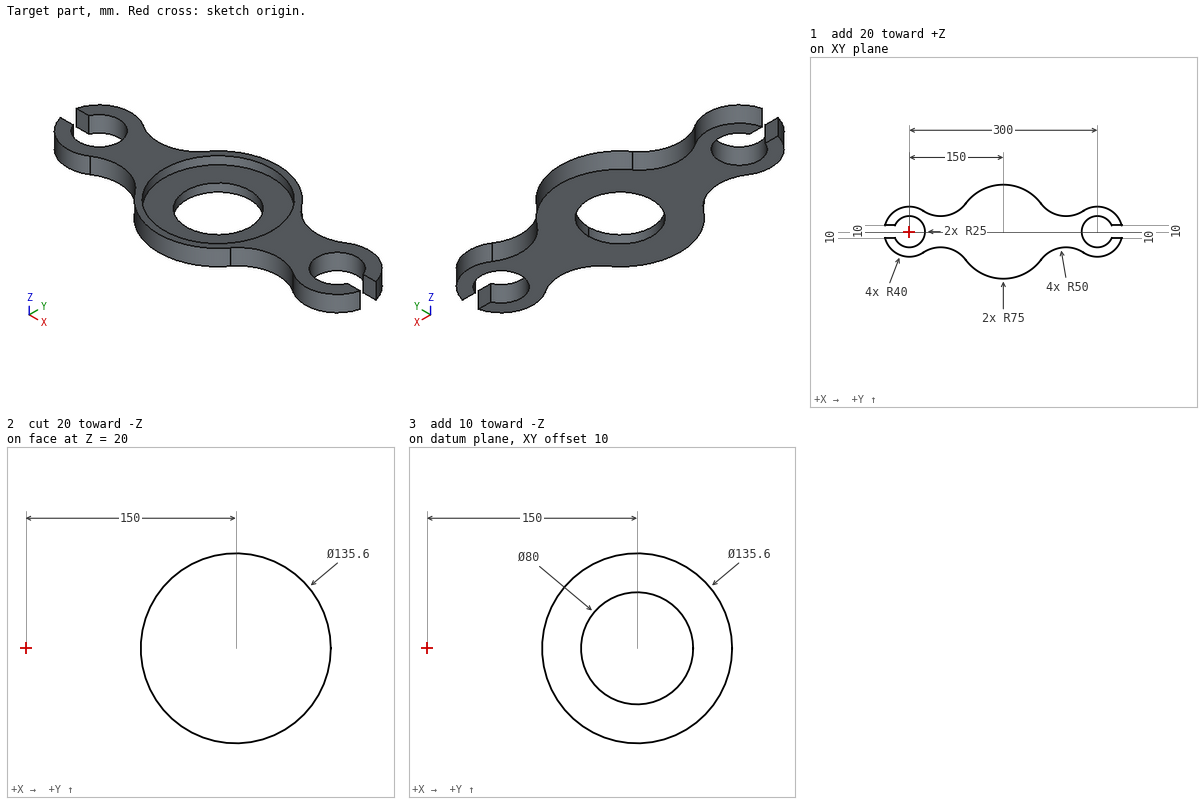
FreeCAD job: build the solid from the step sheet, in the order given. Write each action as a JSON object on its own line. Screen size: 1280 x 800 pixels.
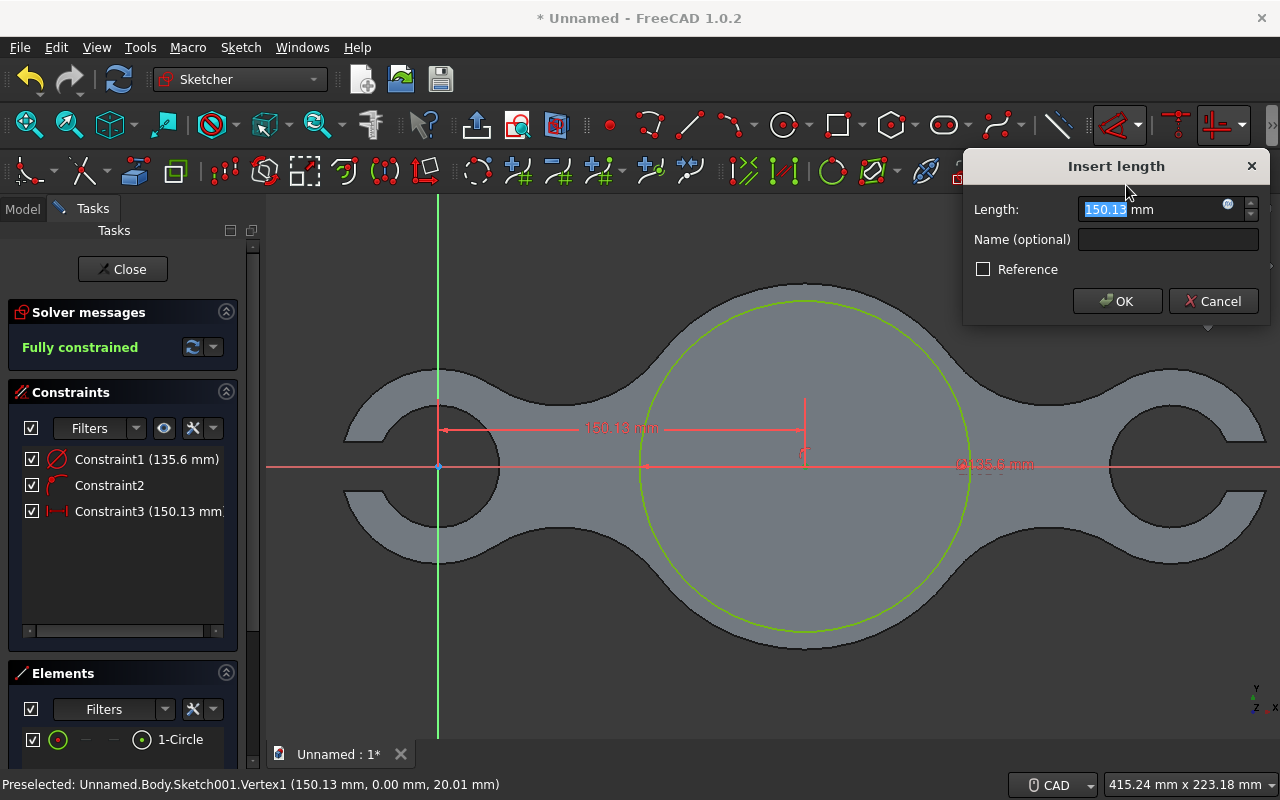
{"action": "type", "text": "150"}
{"action": "key", "text": "Return"}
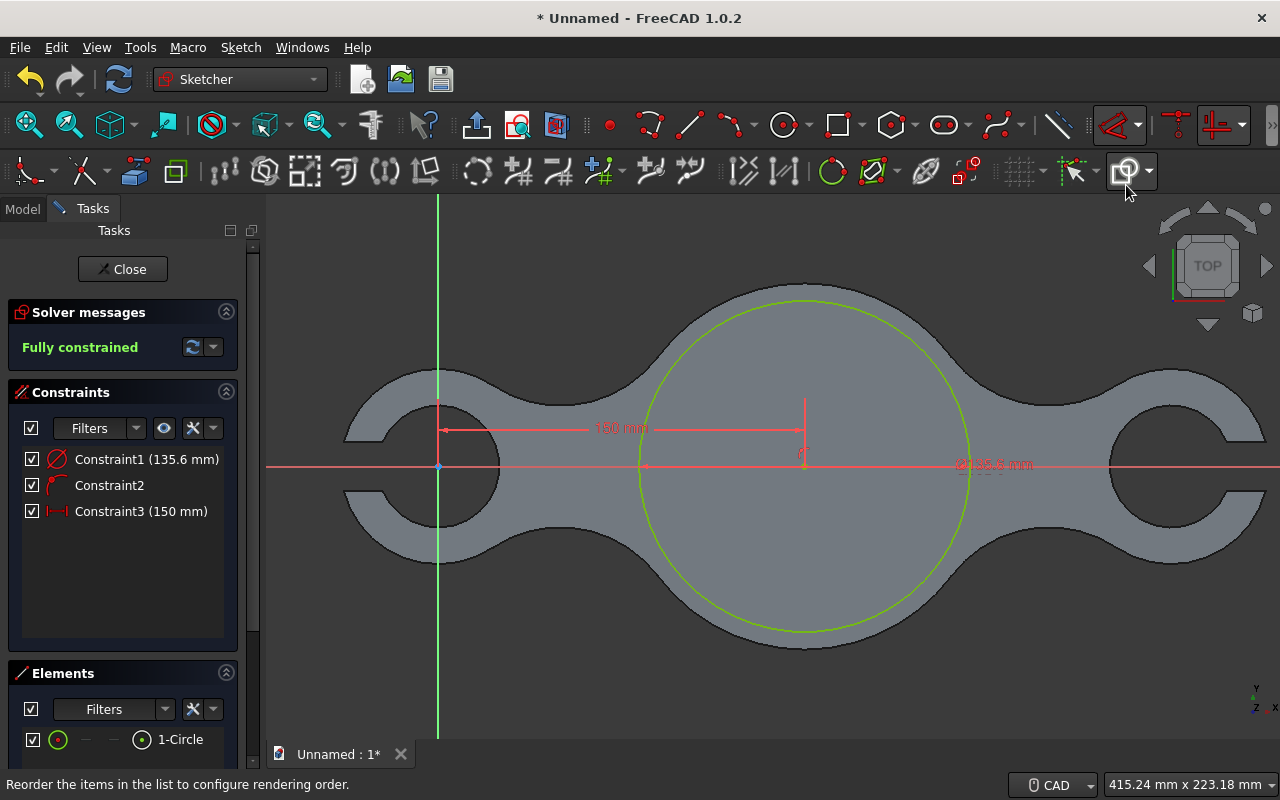
{"action": "left_click", "coordinate": [123, 269]}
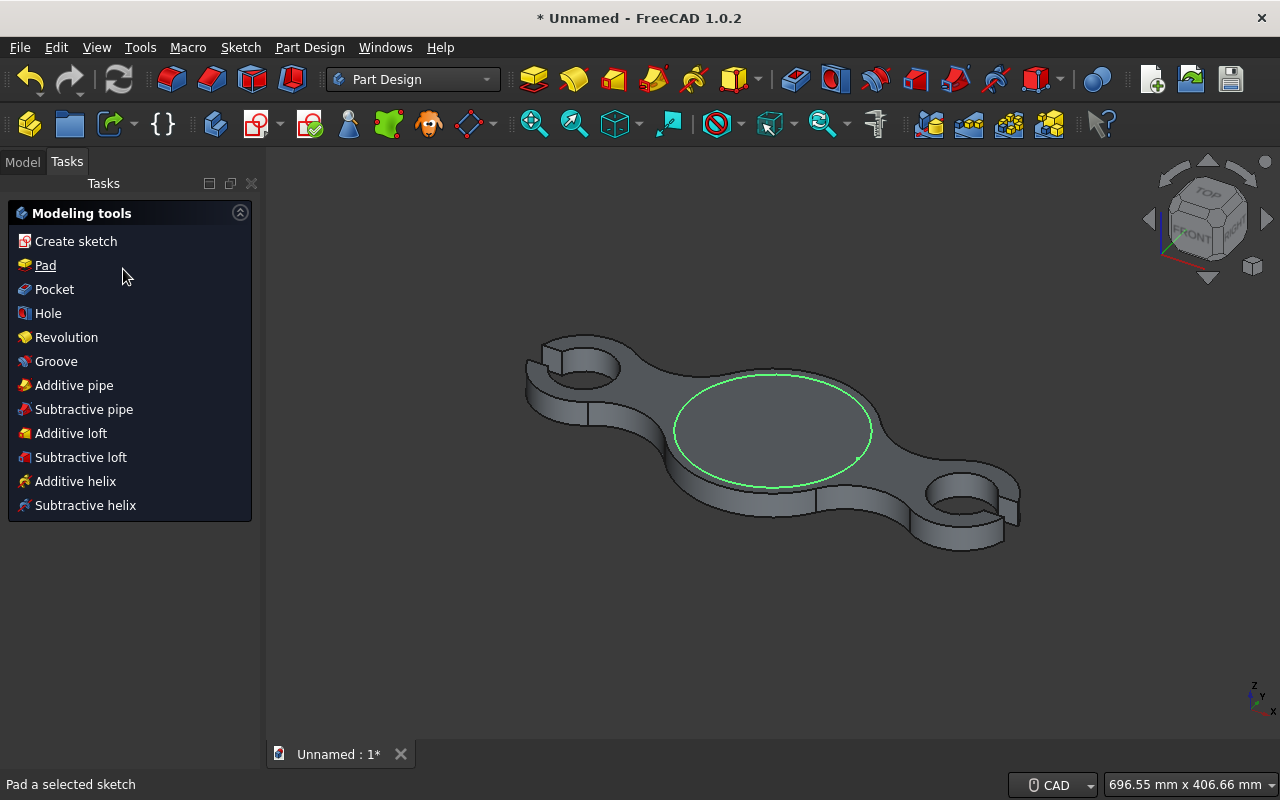
{"action": "left_click", "coordinate": [796, 80]}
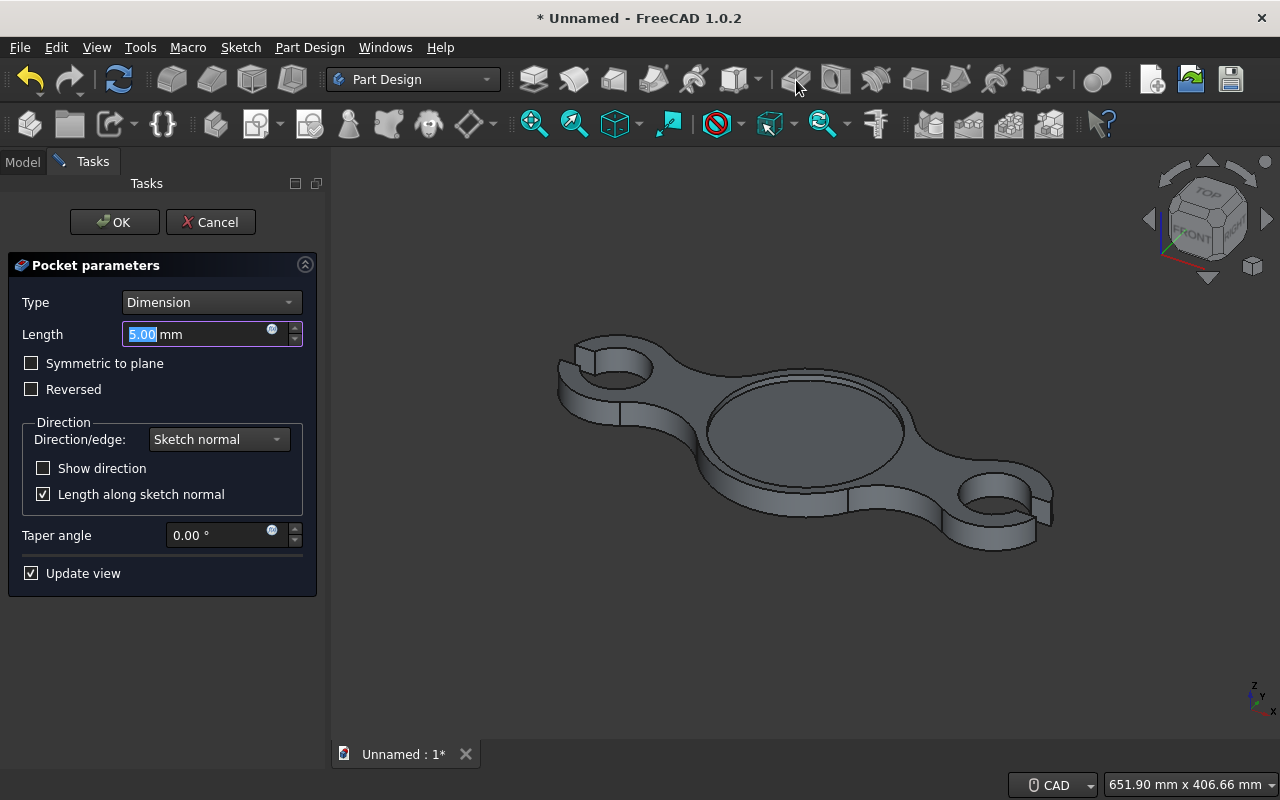
{"action": "type", "text": "20"}
{"action": "key", "text": "Tab"}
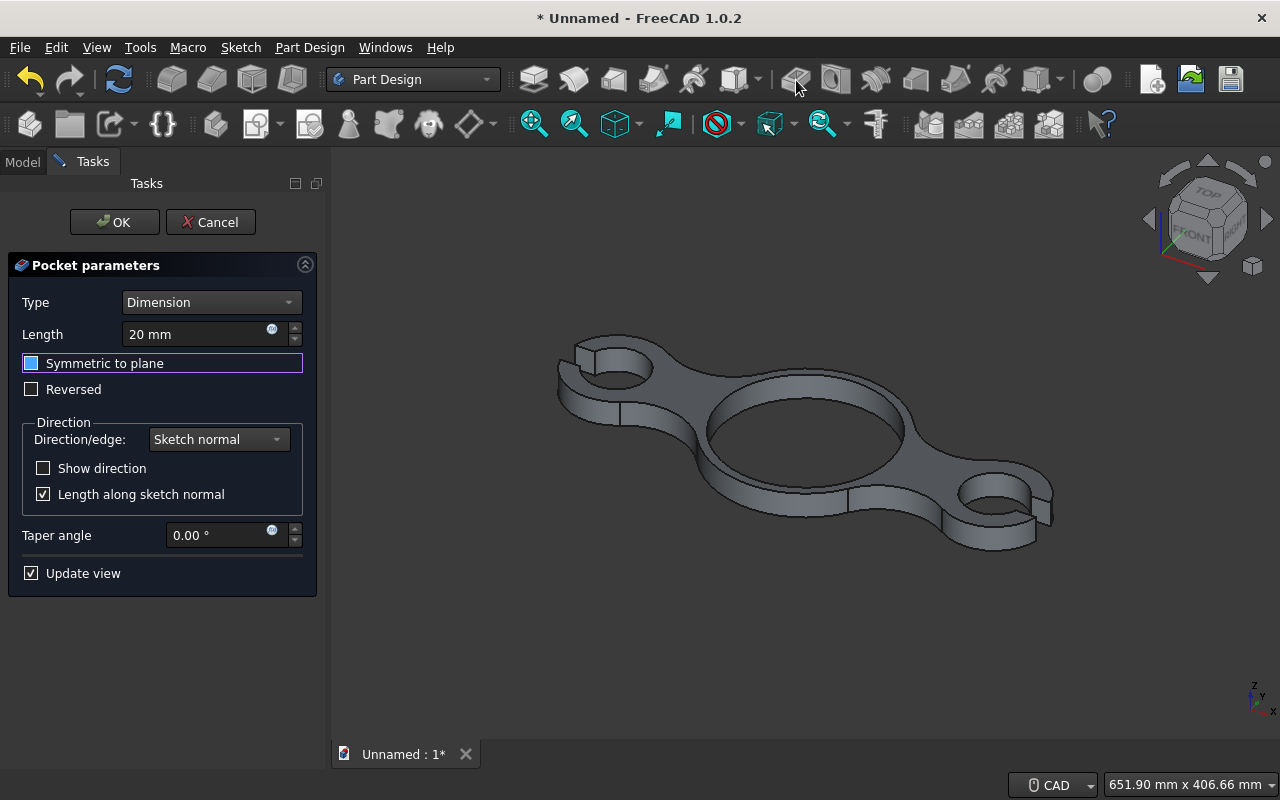
{"action": "left_click", "coordinate": [115, 222]}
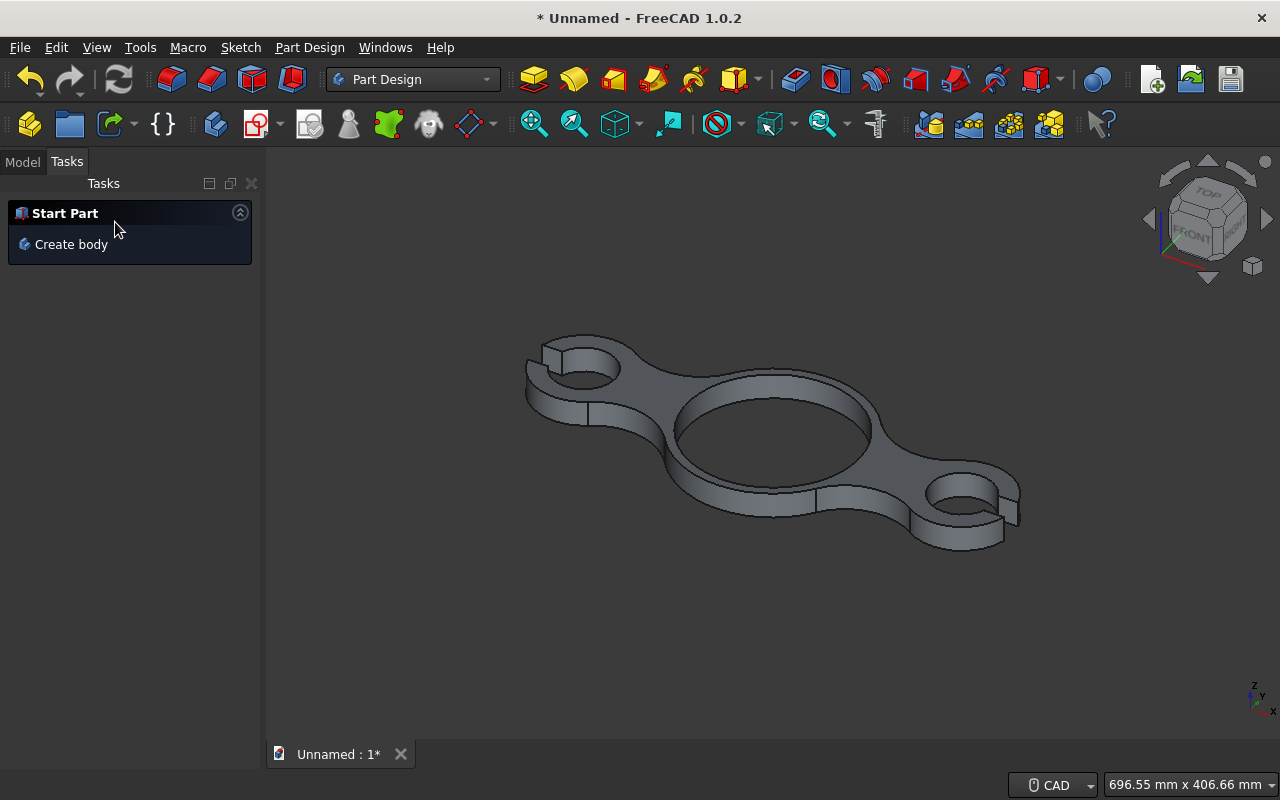
{"action": "left_click", "coordinate": [23, 161]}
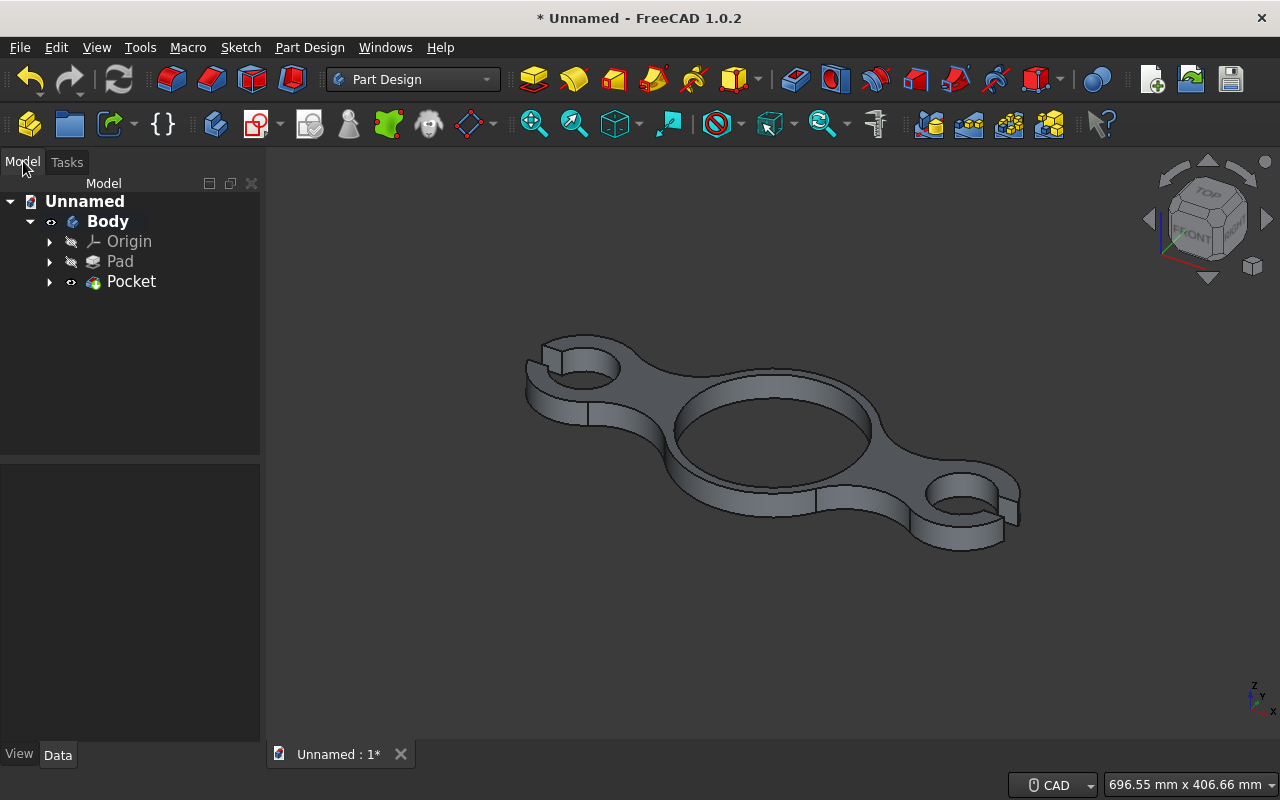
{"action": "left_click", "coordinate": [50, 242]}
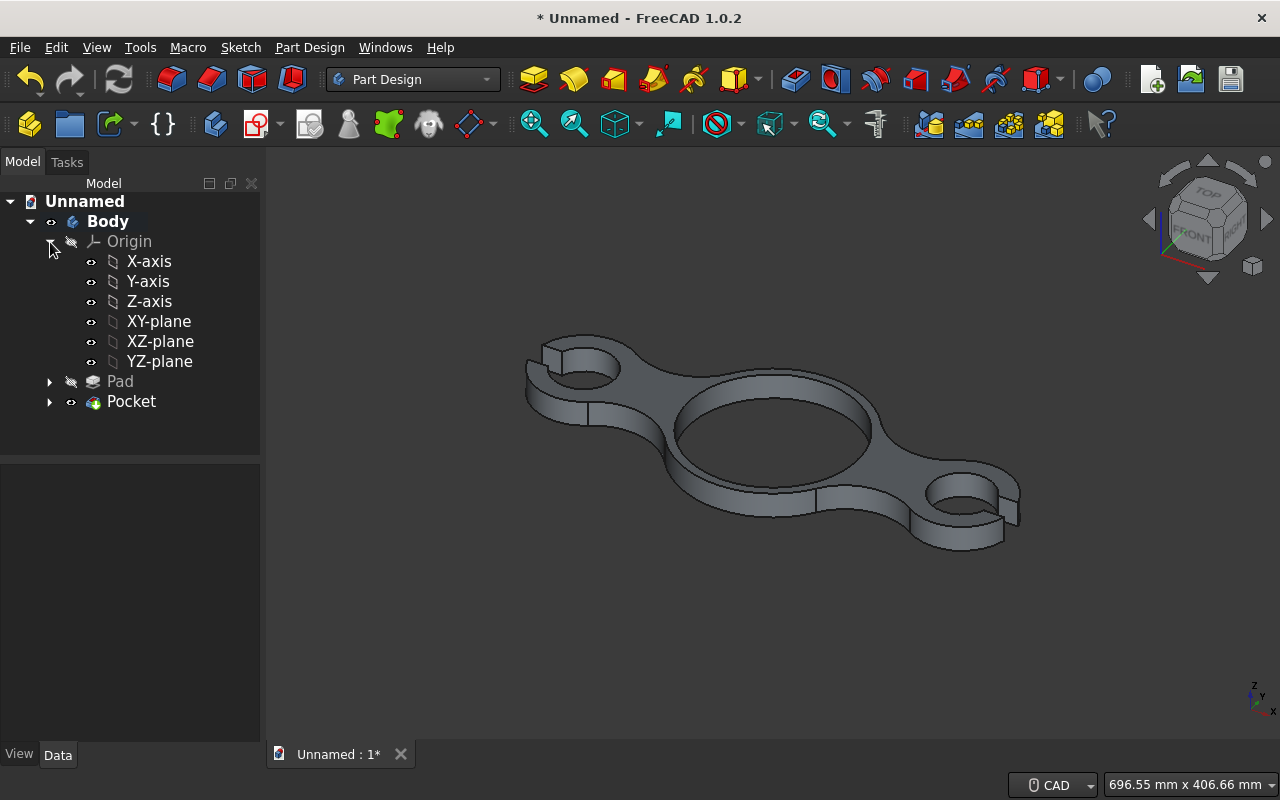
{"action": "left_click", "coordinate": [136, 322]}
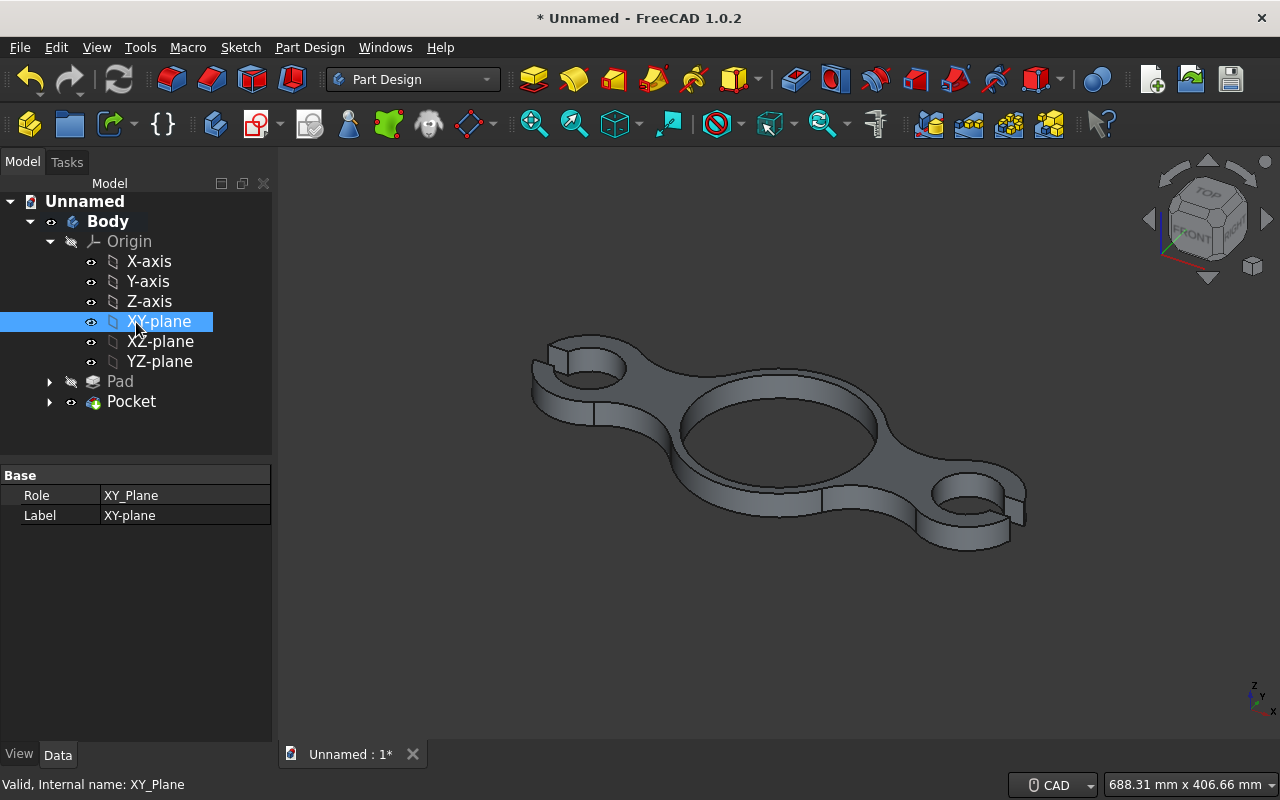
{"action": "left_click", "coordinate": [470, 124]}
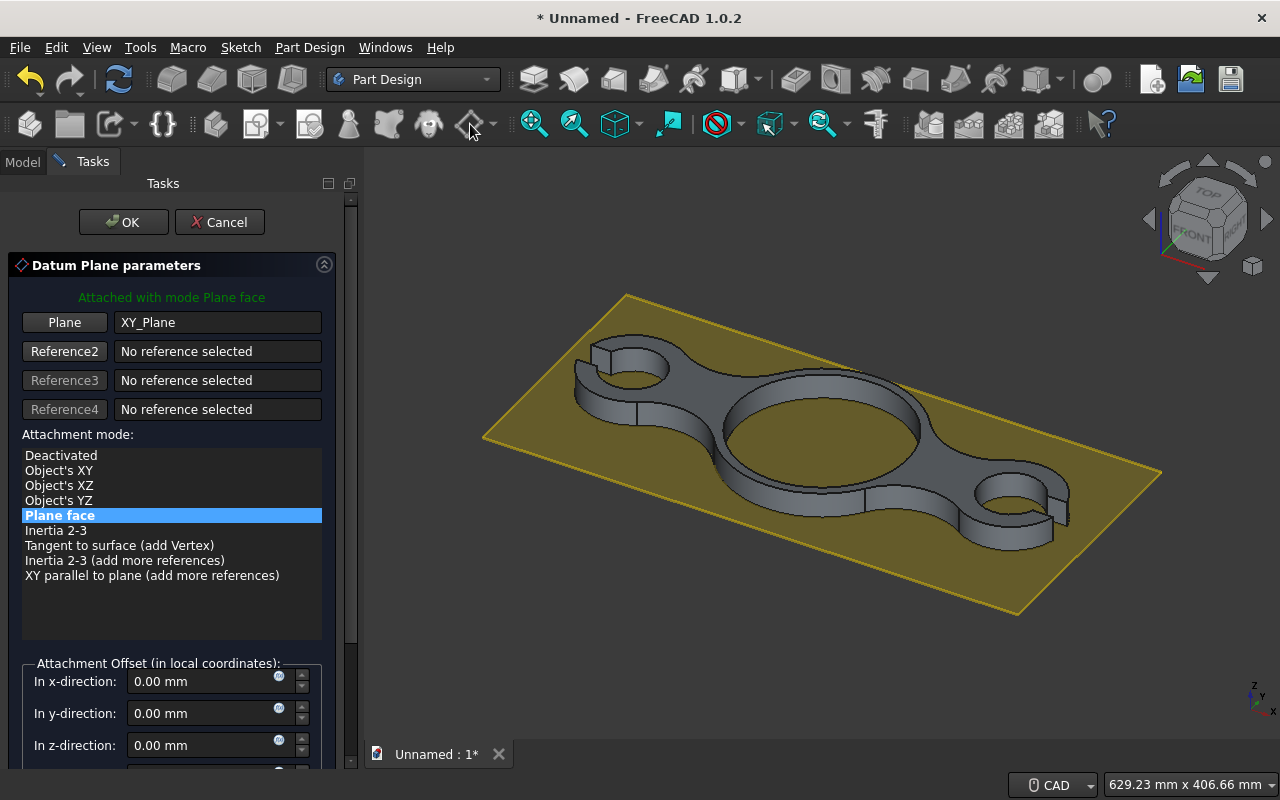
{"action": "triple_click", "coordinate": [210, 745]}